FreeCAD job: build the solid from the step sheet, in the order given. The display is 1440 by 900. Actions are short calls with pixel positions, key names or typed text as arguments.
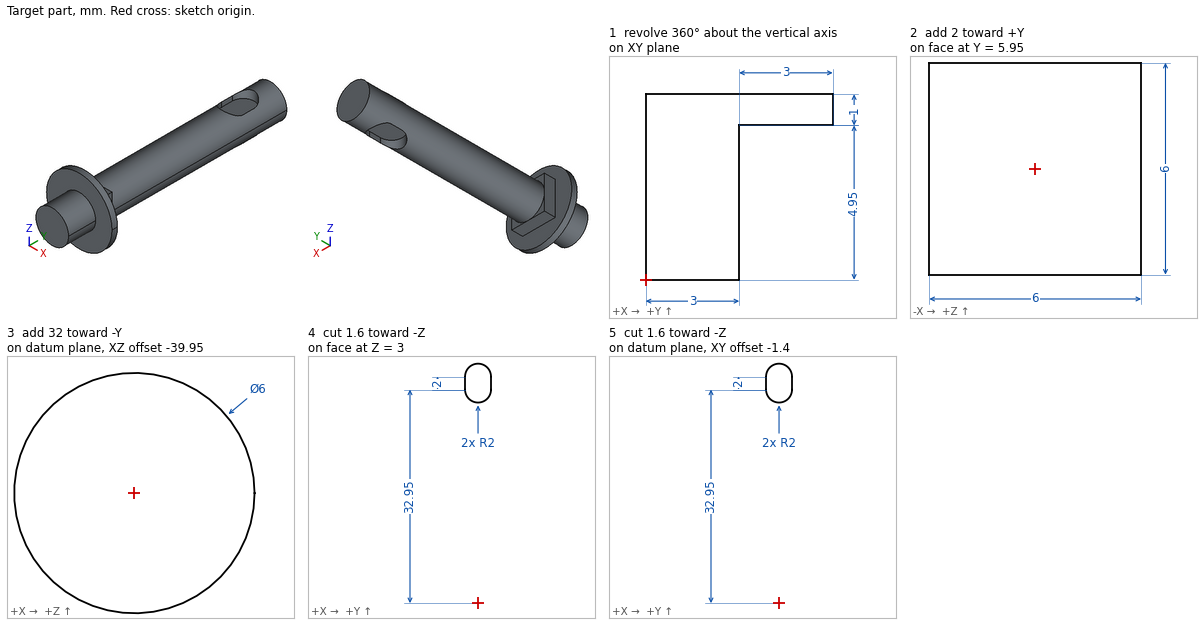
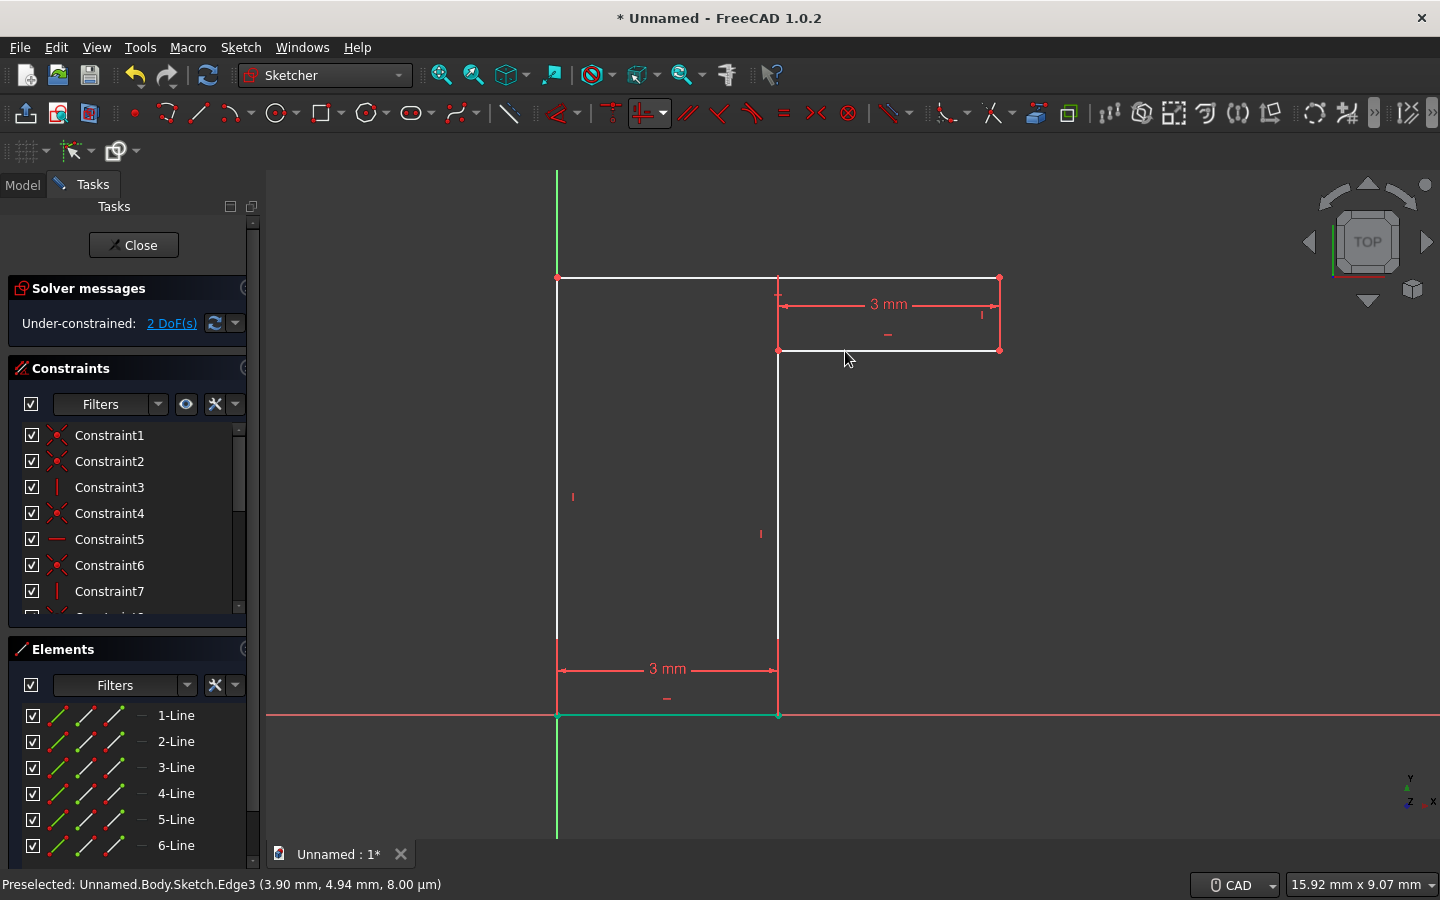
click(1000, 329)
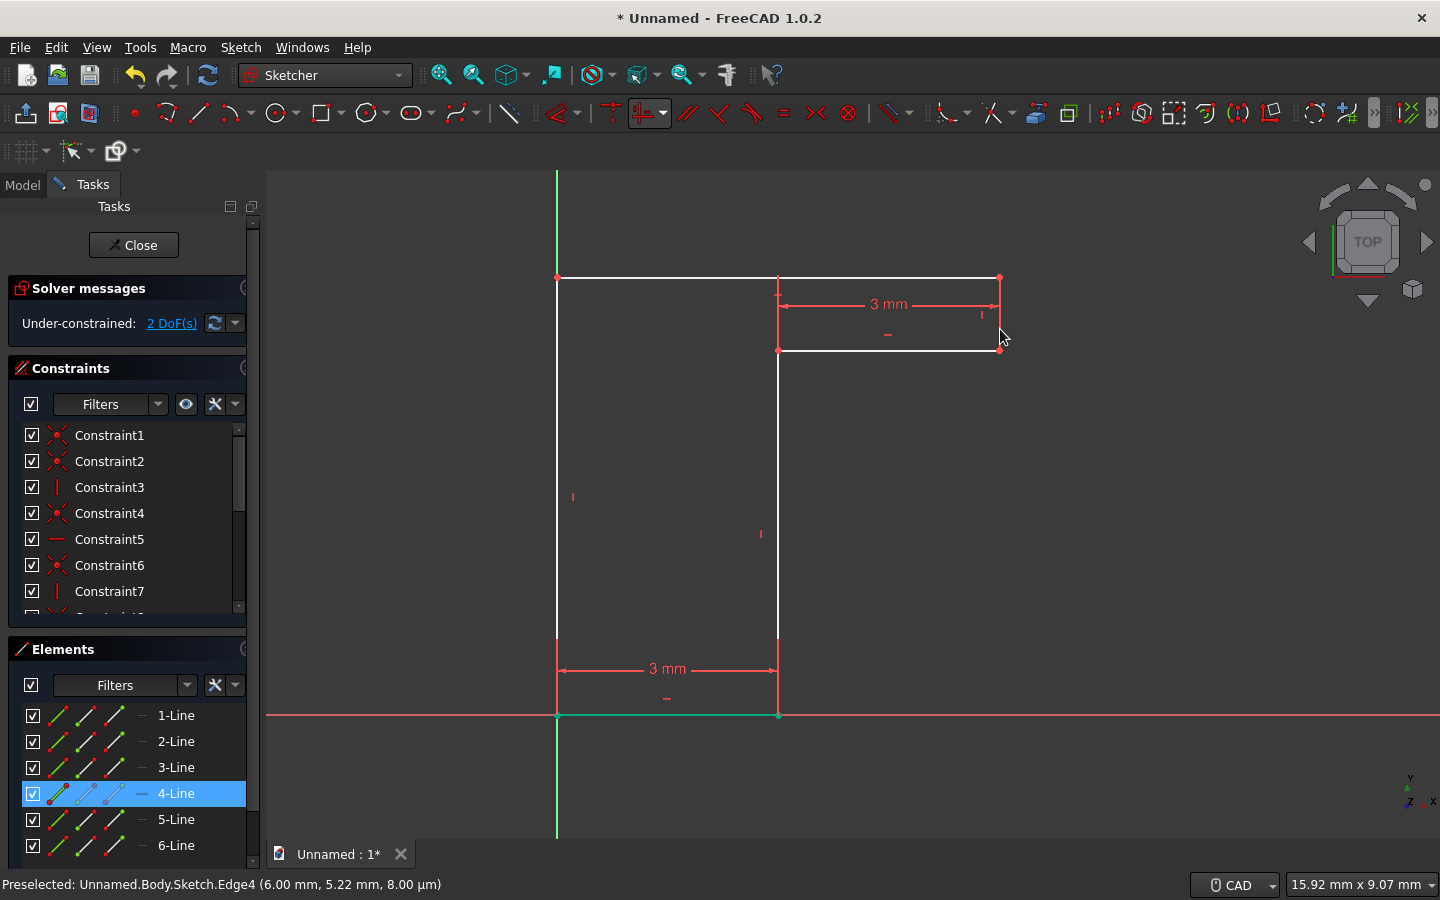
key(i)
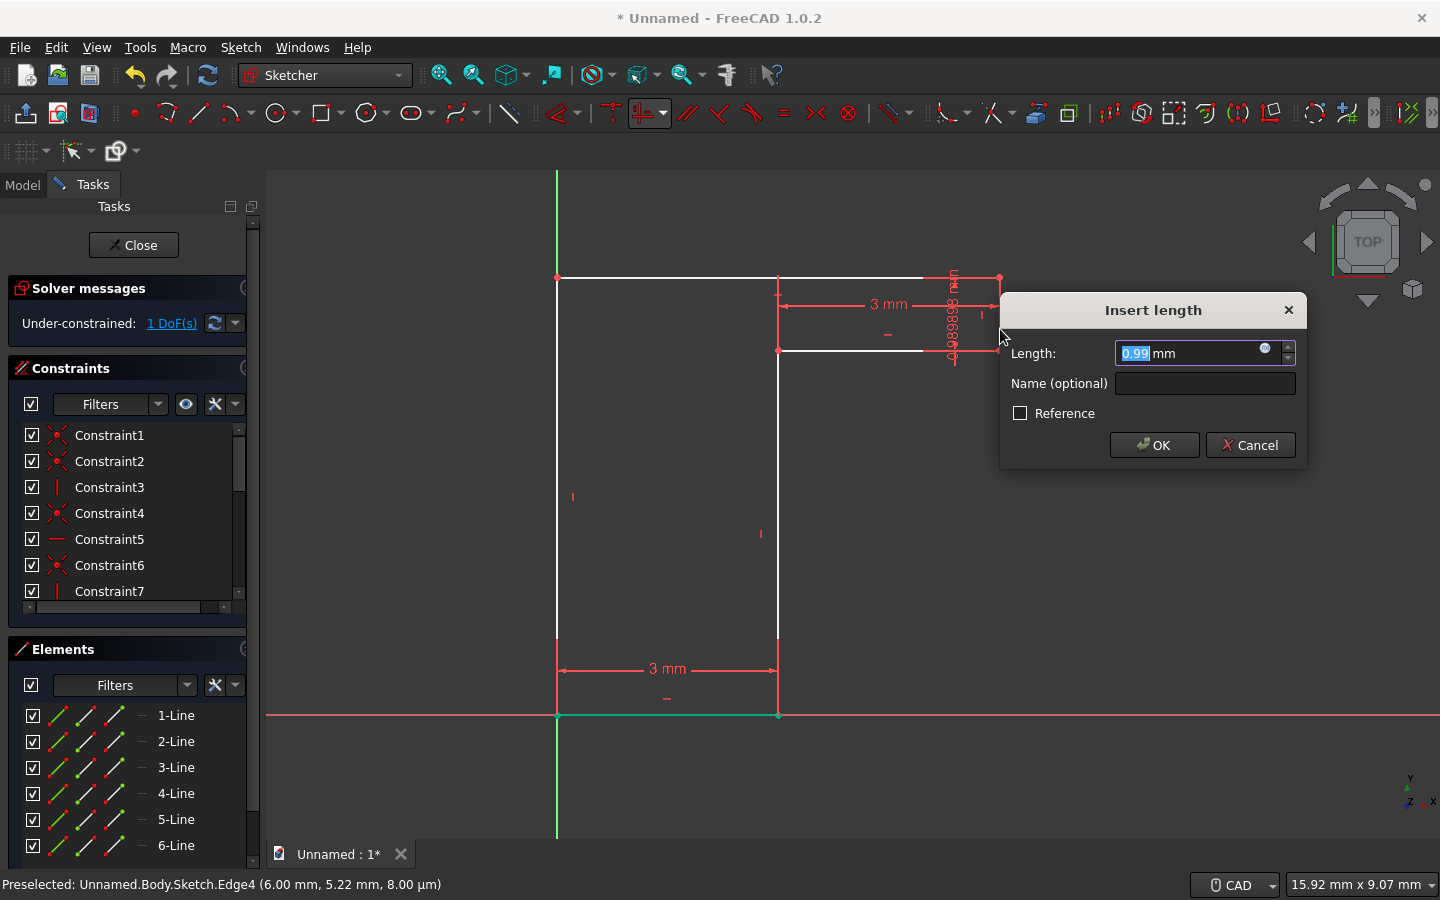
text(1)
key(Return)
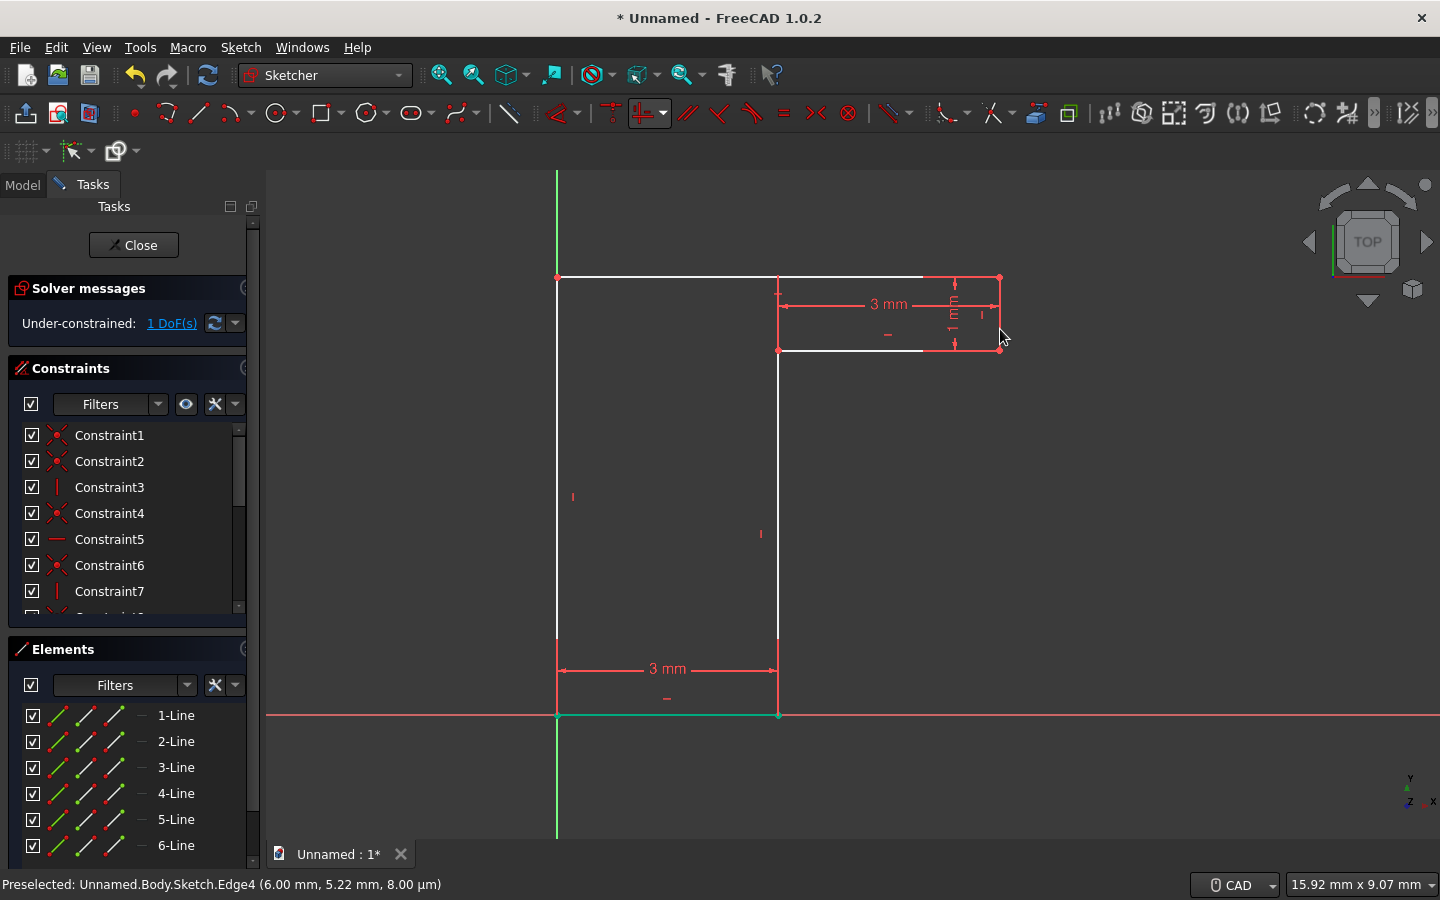
click(778, 606)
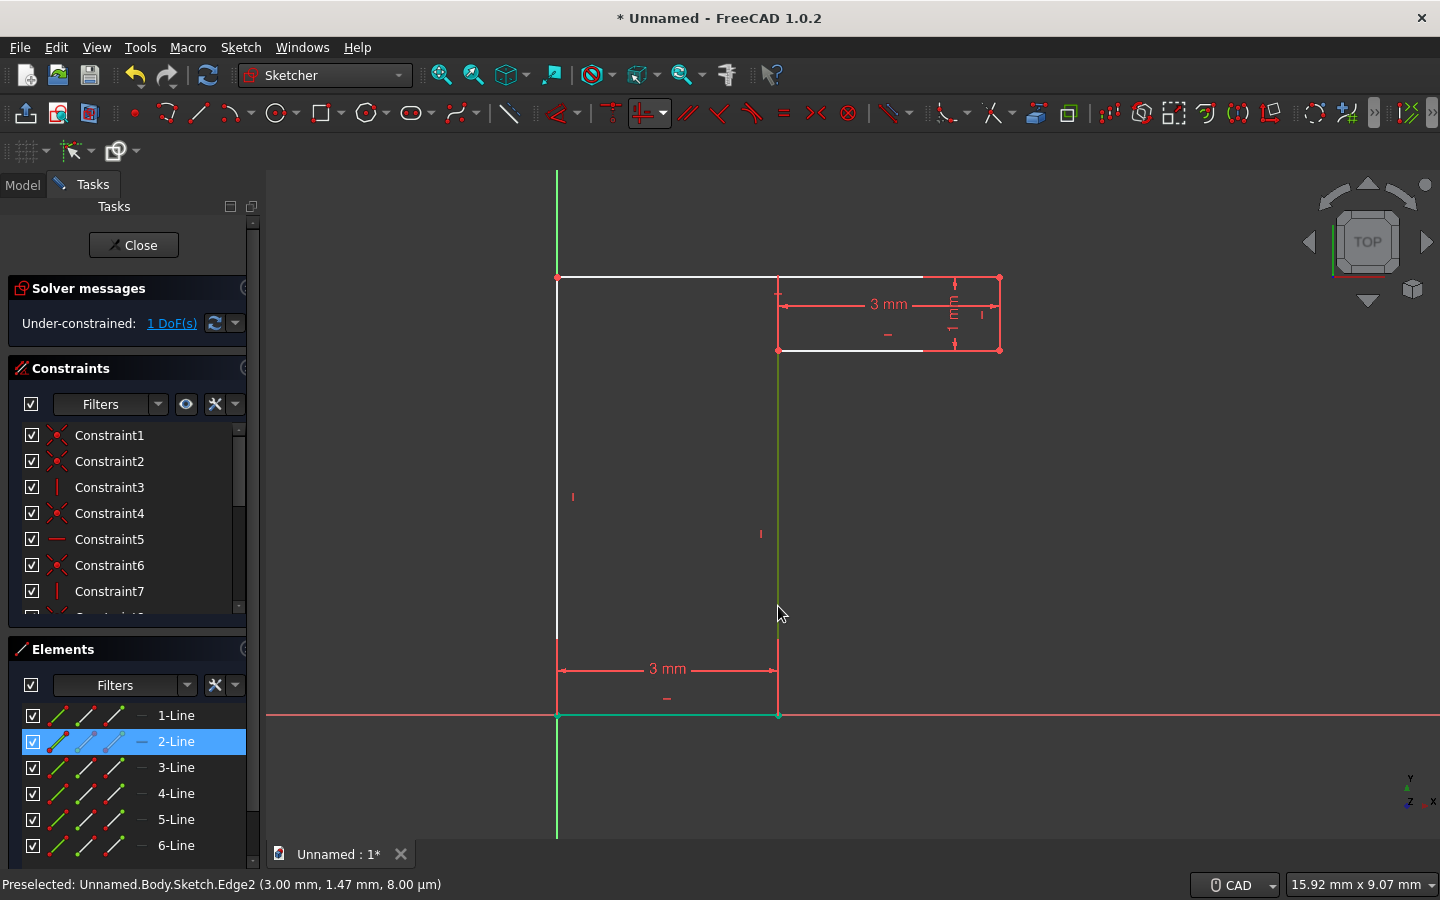
click(580, 114)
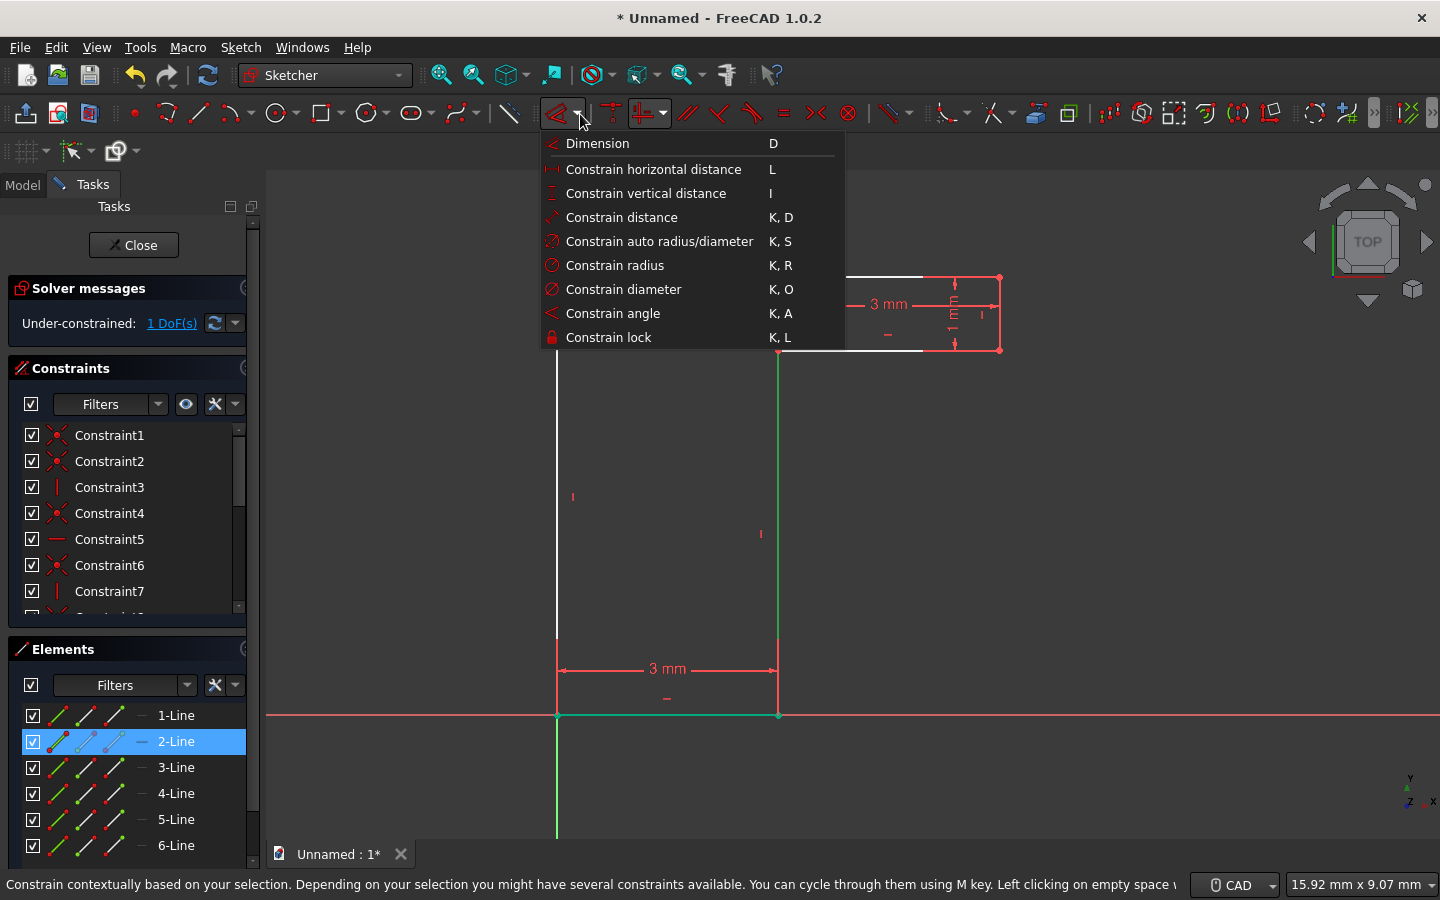
click(693, 193)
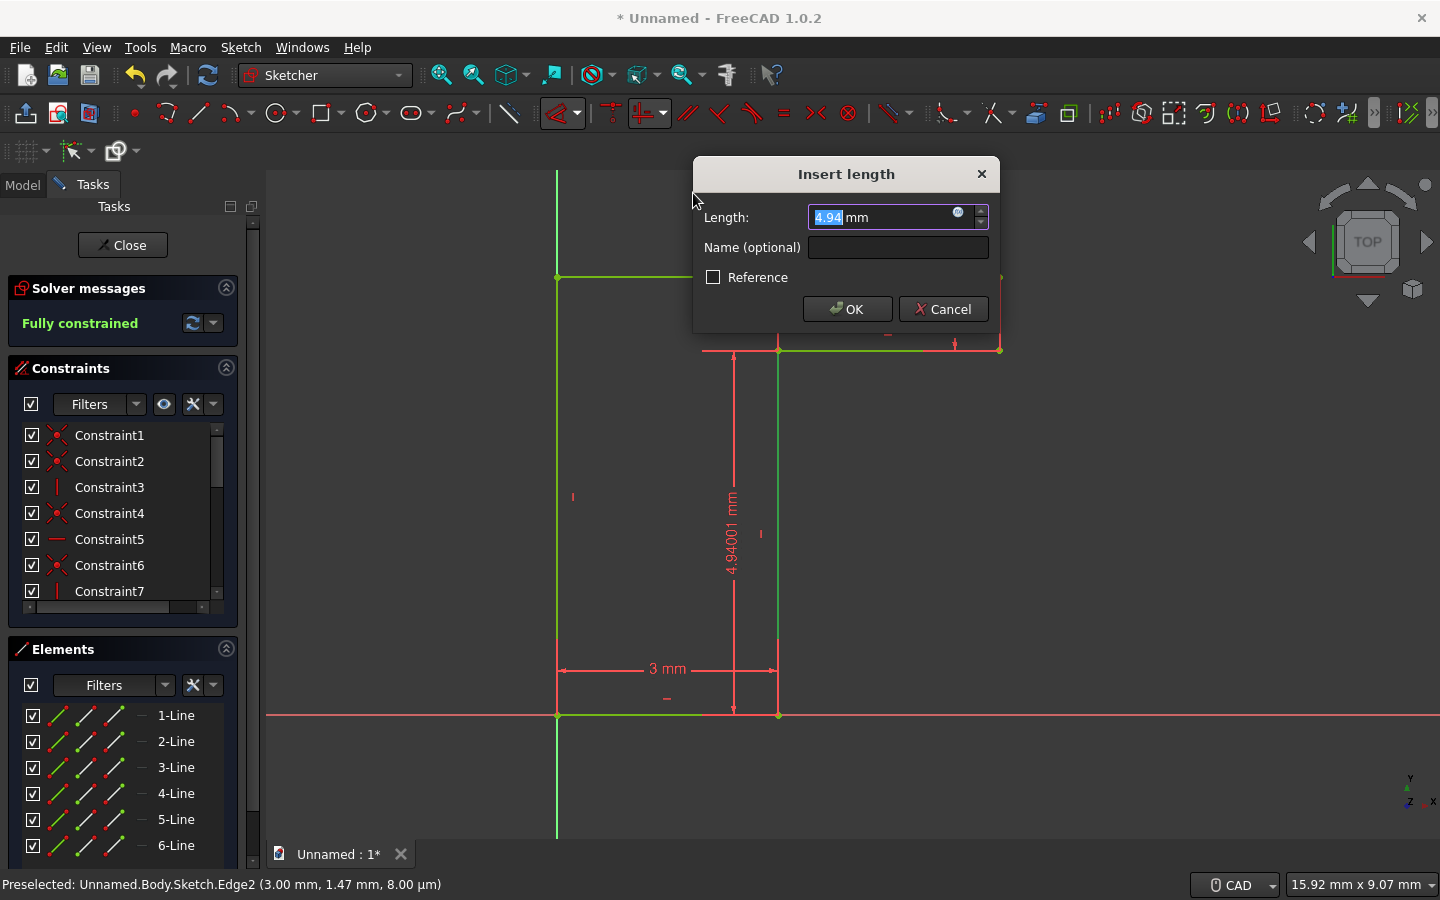
text(4.95)
key(Return)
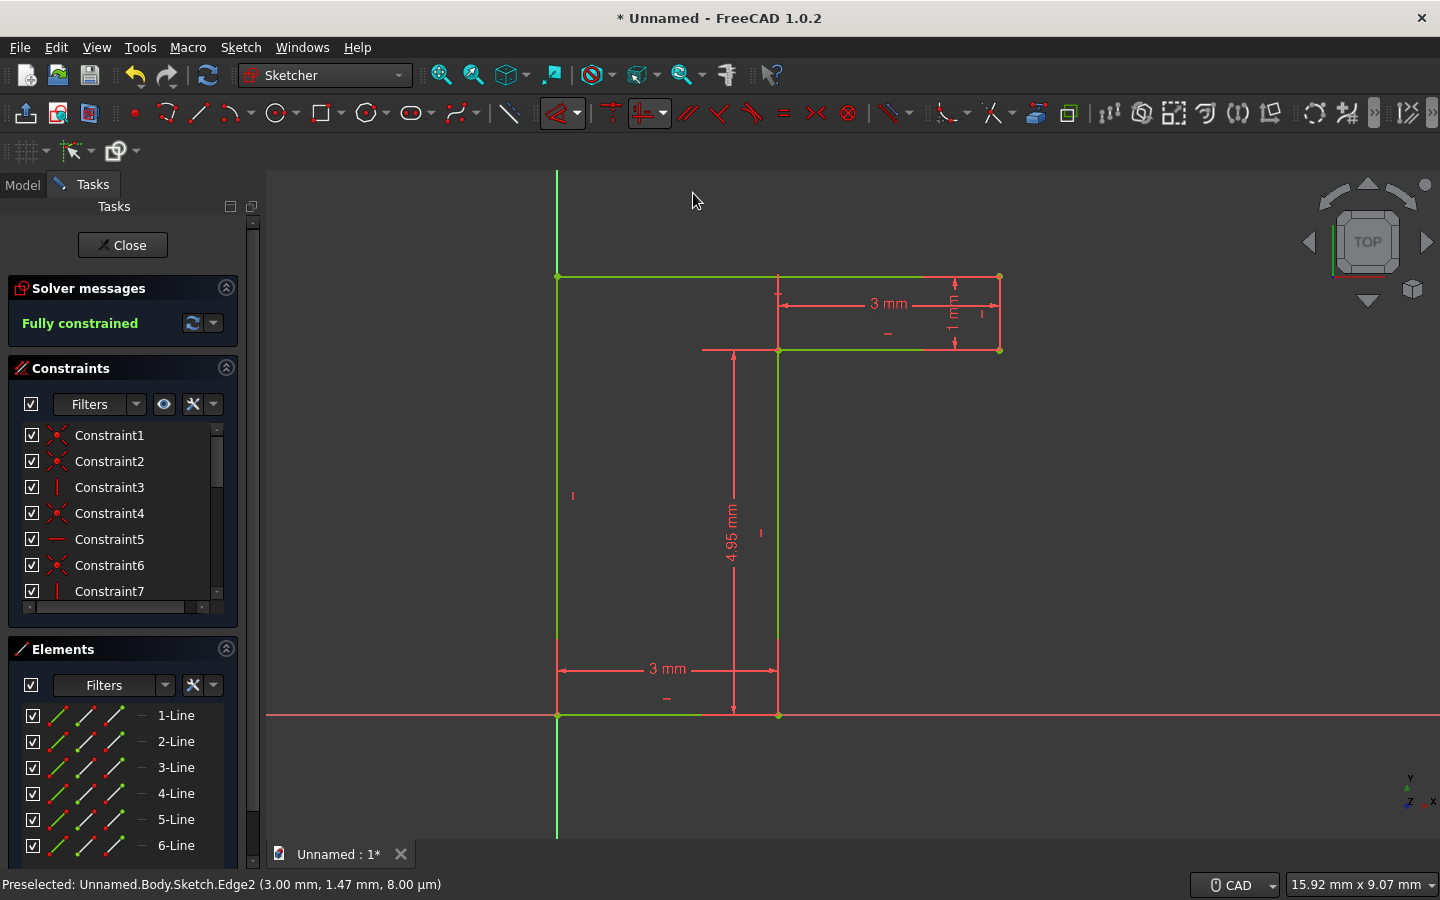
click(123, 245)